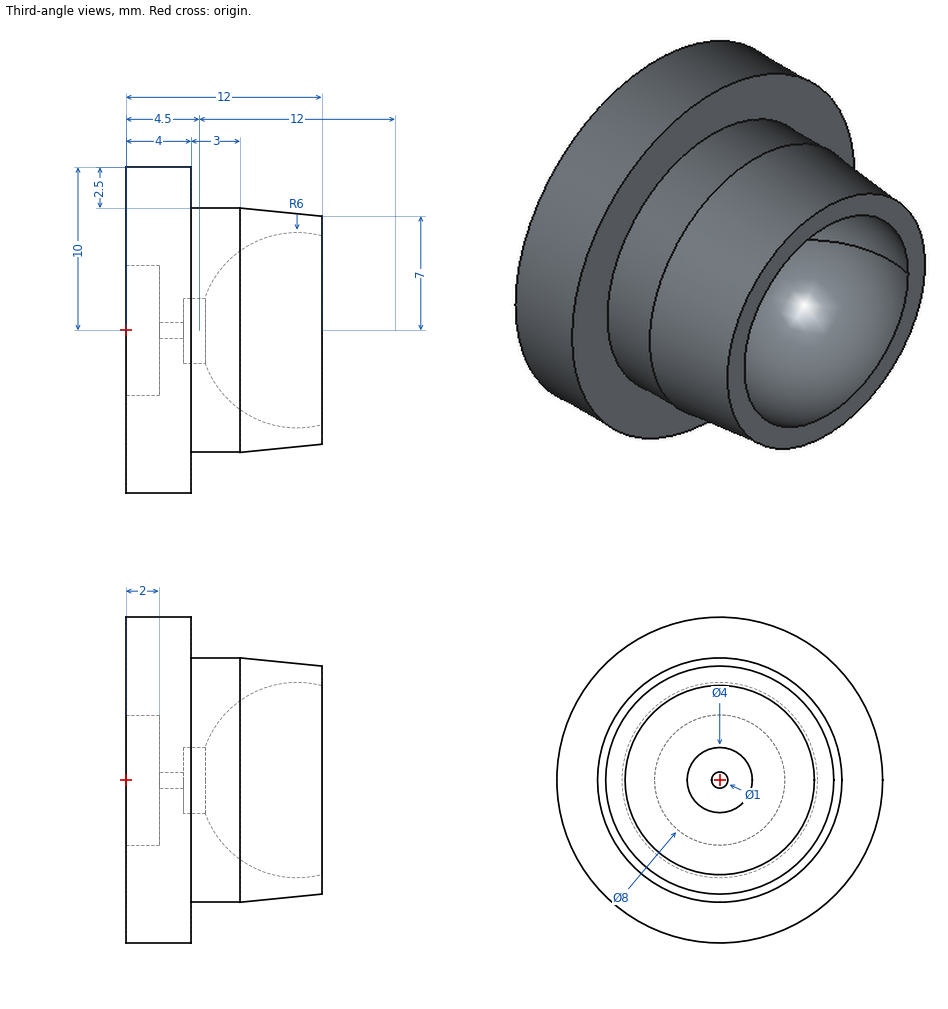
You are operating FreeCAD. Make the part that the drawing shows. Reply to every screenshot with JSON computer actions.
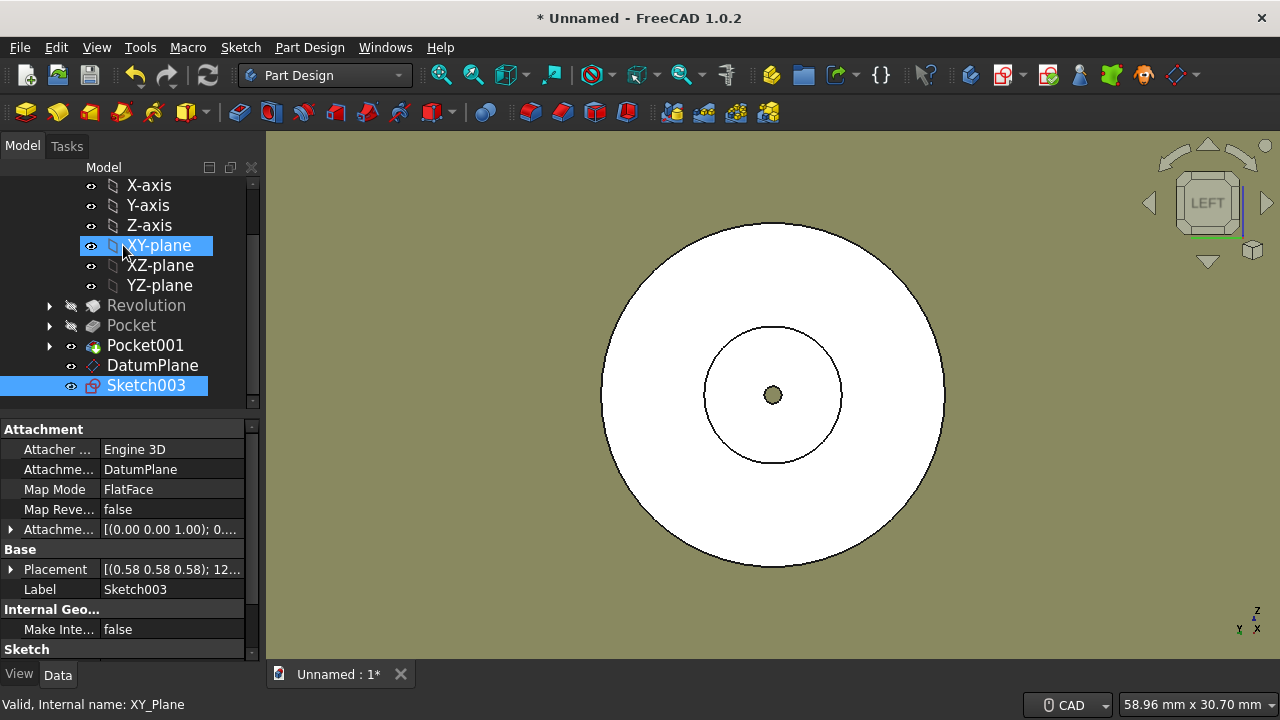
{"action": "left_click", "coordinate": [240, 112]}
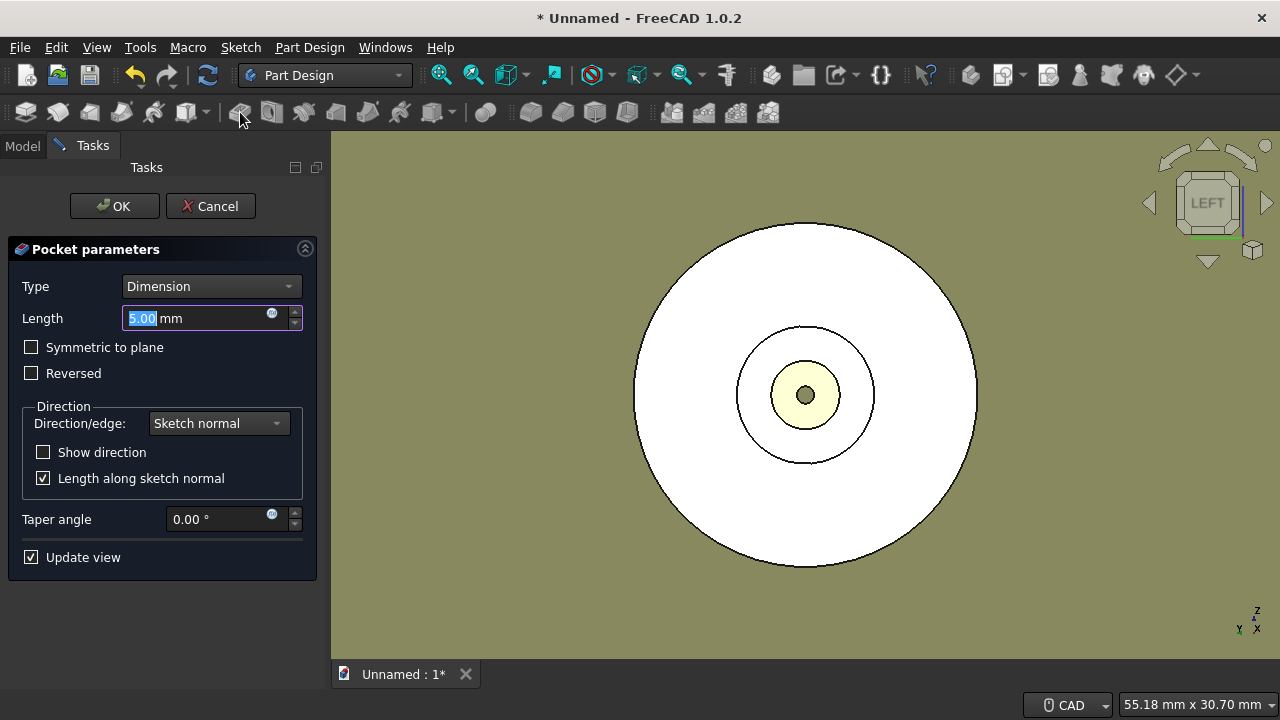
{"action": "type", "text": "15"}
{"action": "key", "text": "Tab"}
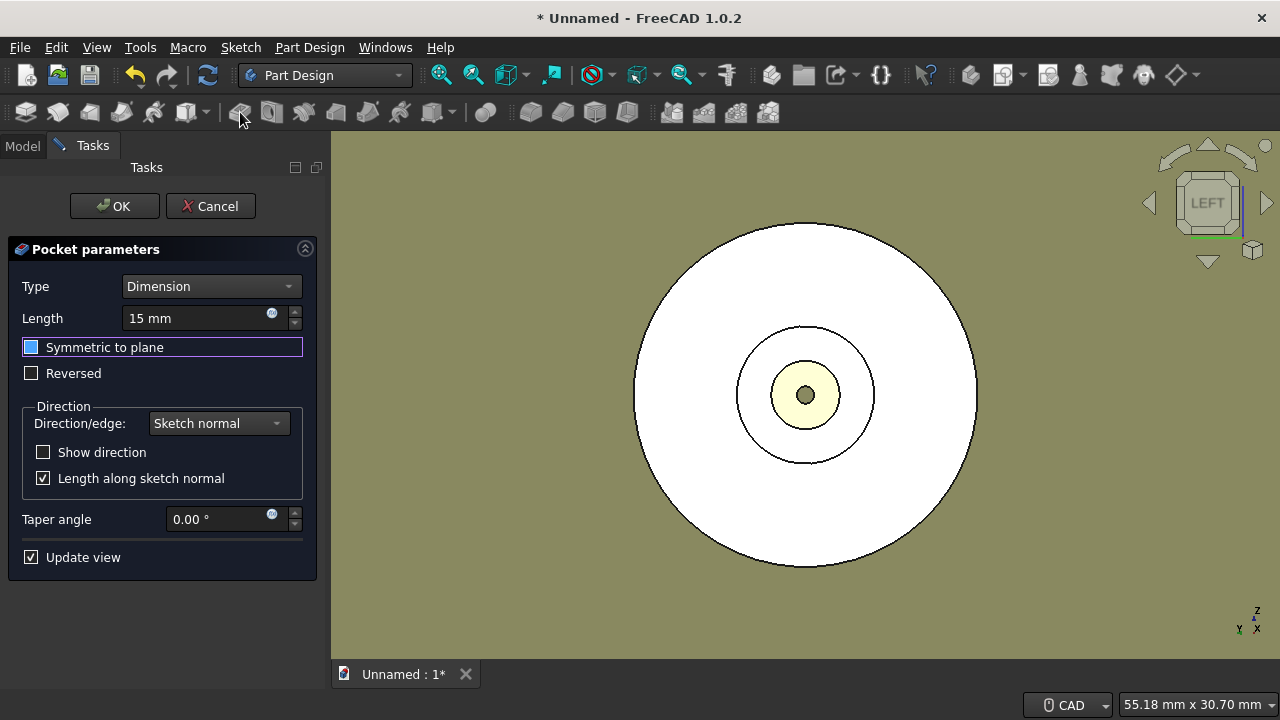
{"action": "left_click", "coordinate": [30, 373]}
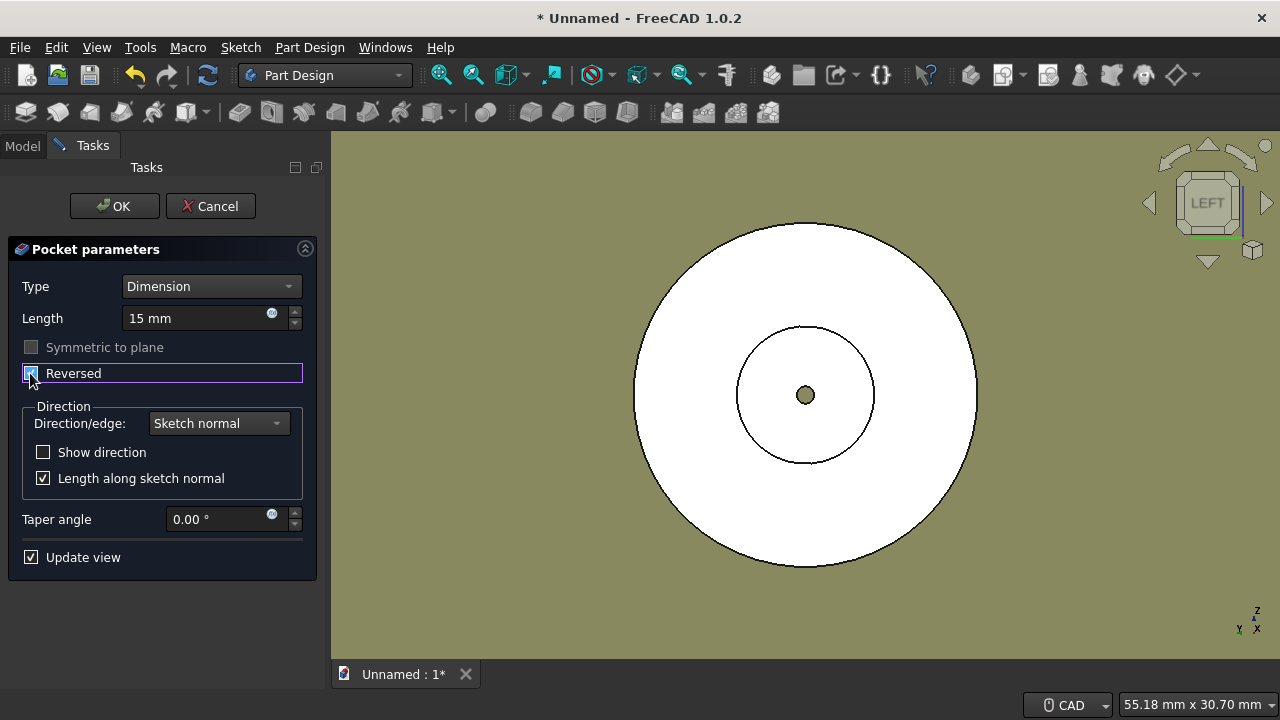
{"action": "left_click", "coordinate": [115, 206]}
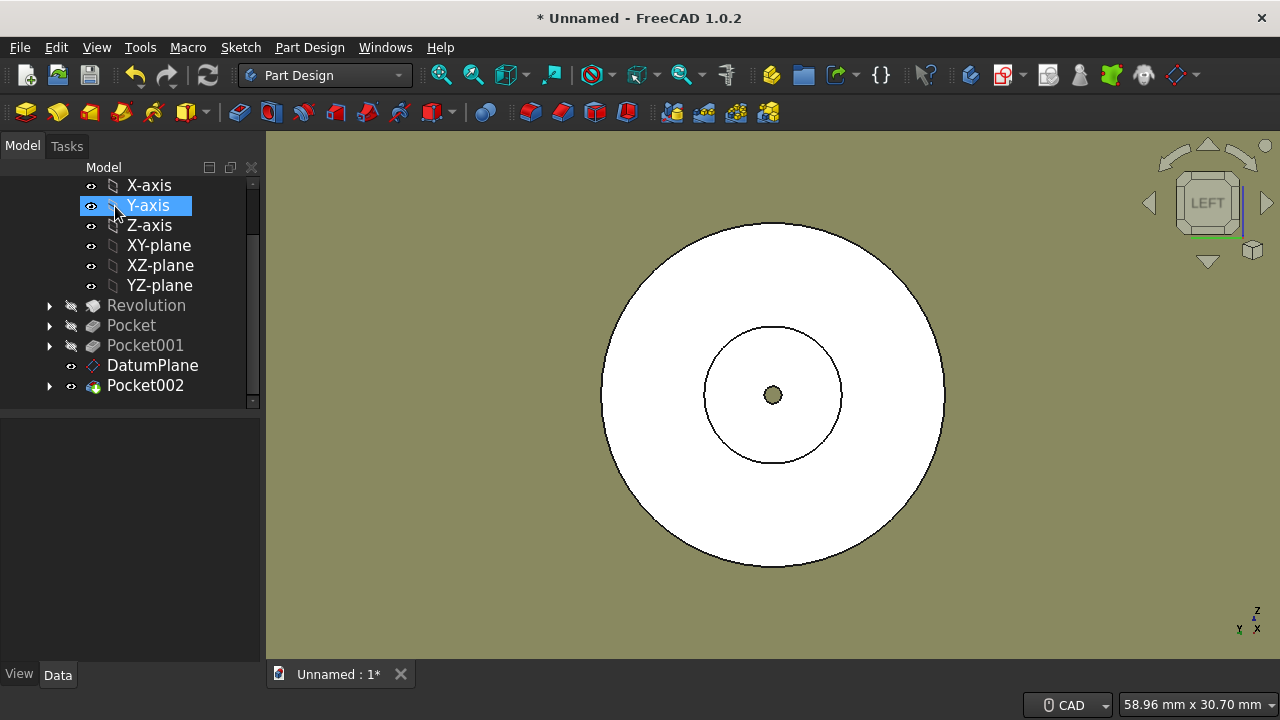
{"action": "left_click", "coordinate": [116, 366]}
{"action": "key", "text": "space"}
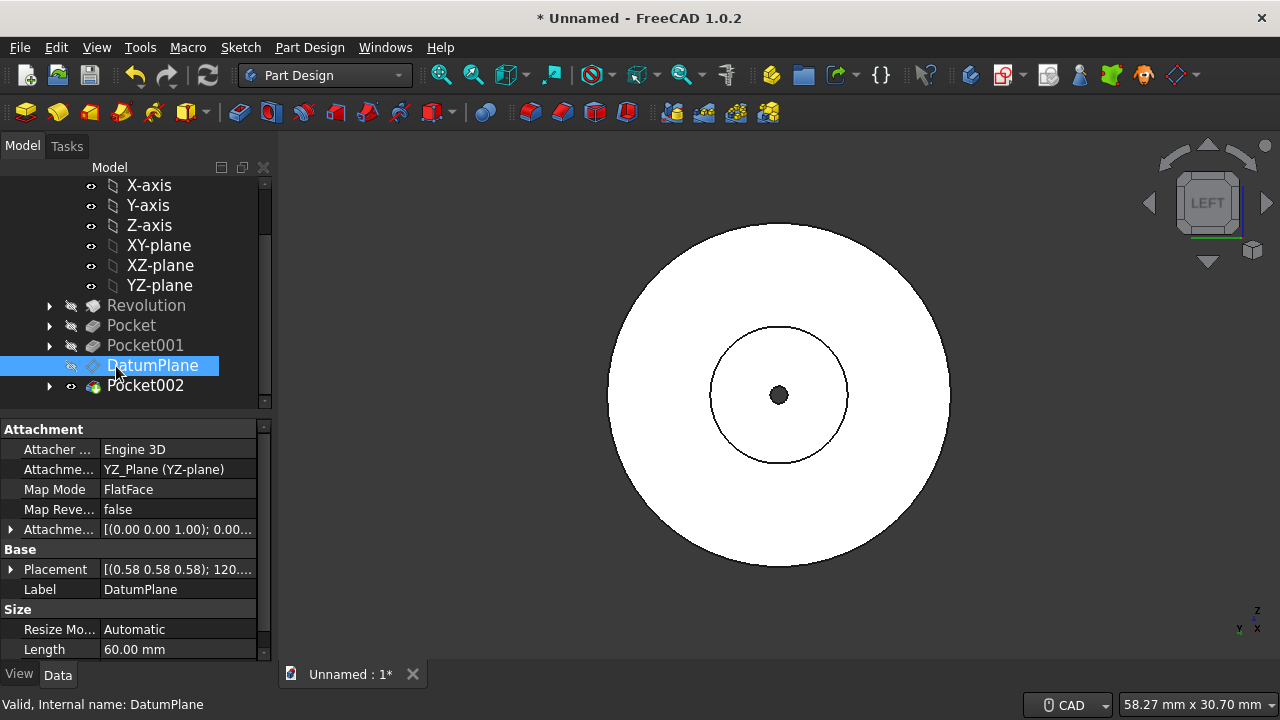
{"action": "left_click", "coordinate": [318, 619]}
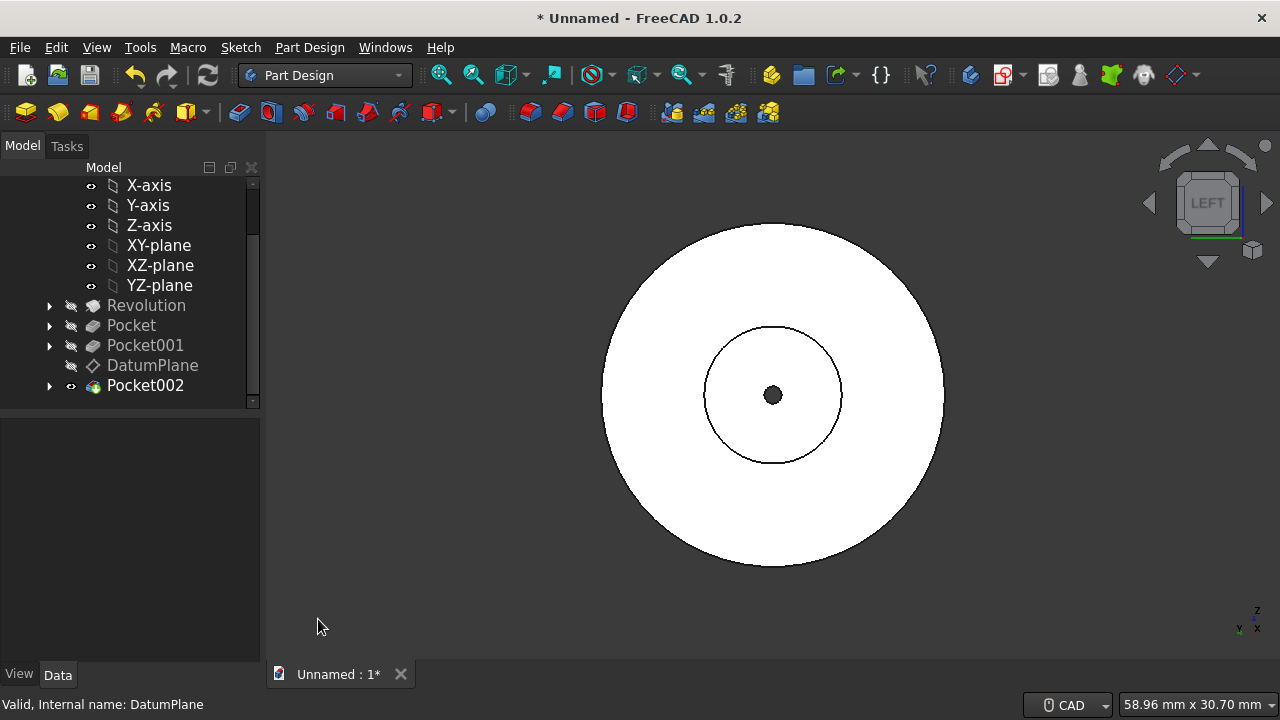
{"action": "left_click", "coordinate": [1004, 76]}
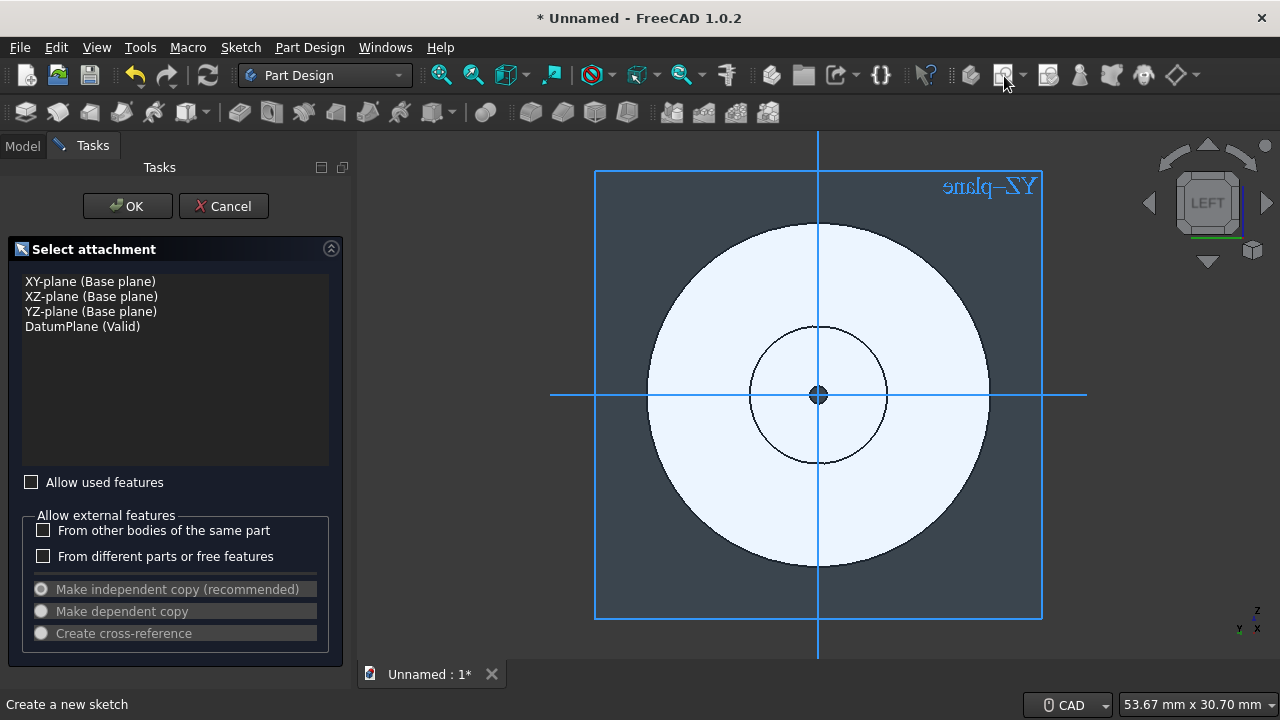
{"action": "left_click", "coordinate": [82, 282]}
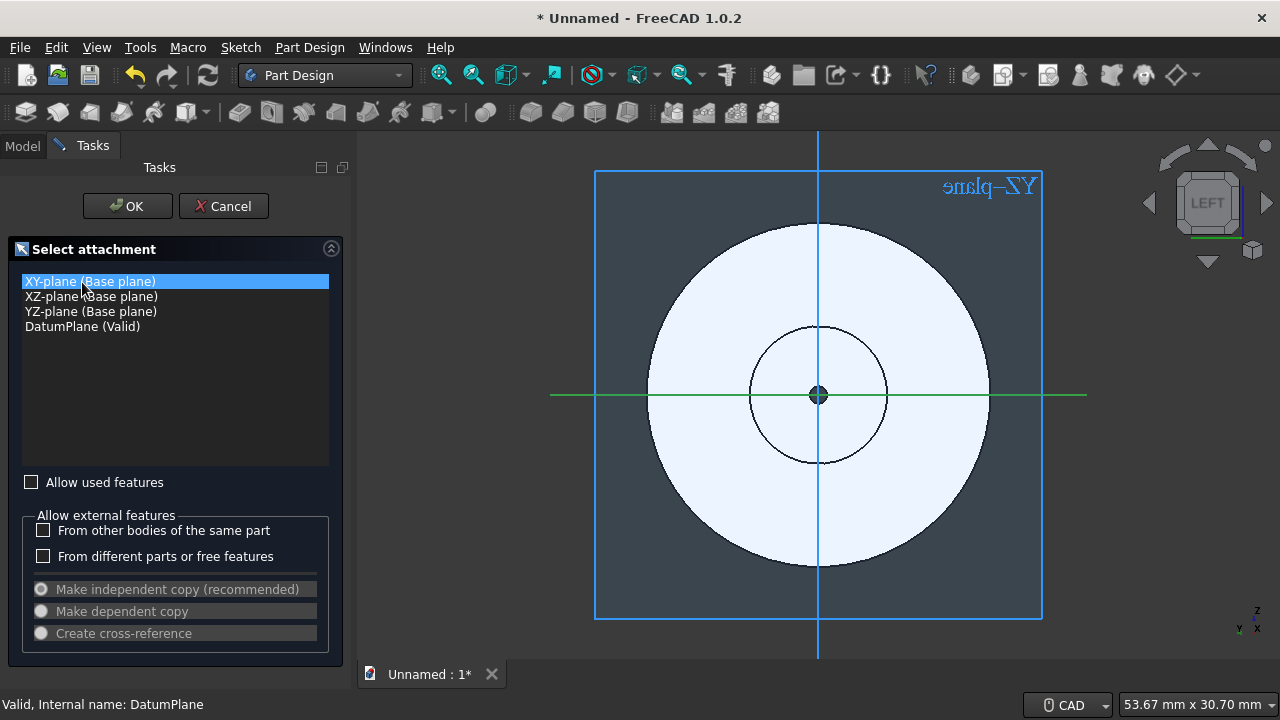
{"action": "left_click", "coordinate": [128, 206]}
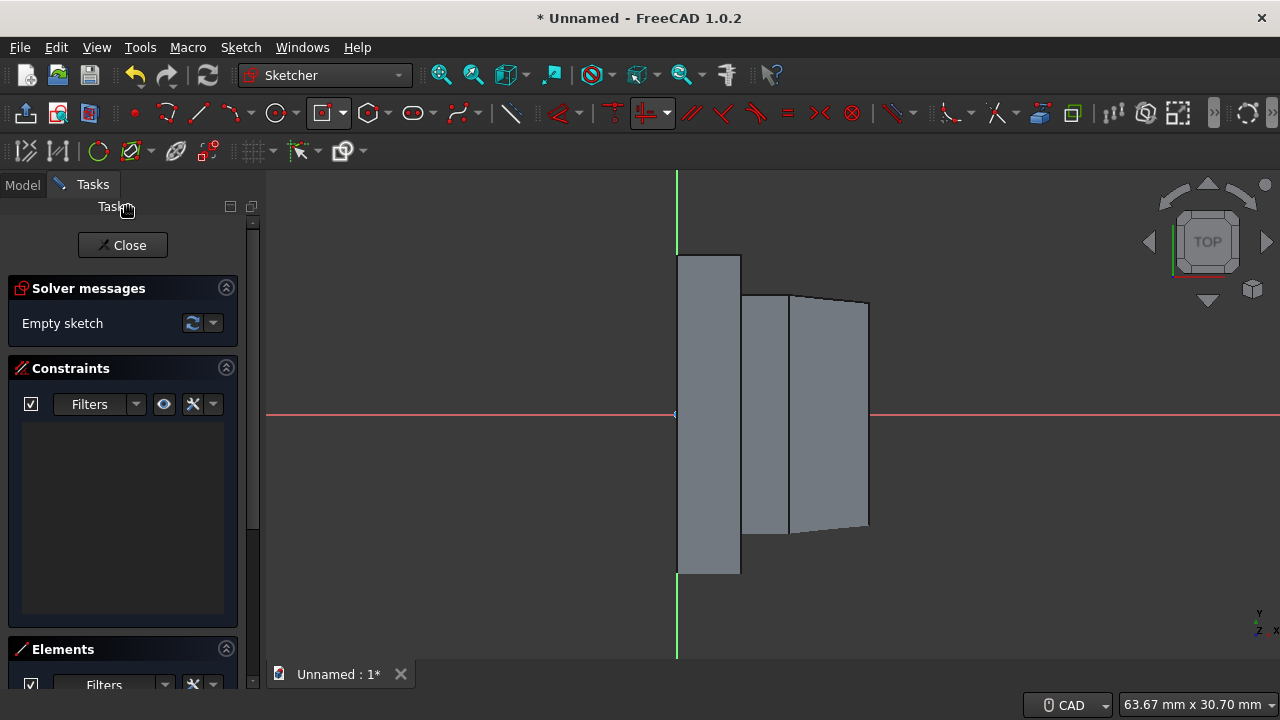
{"action": "left_click", "coordinate": [90, 114]}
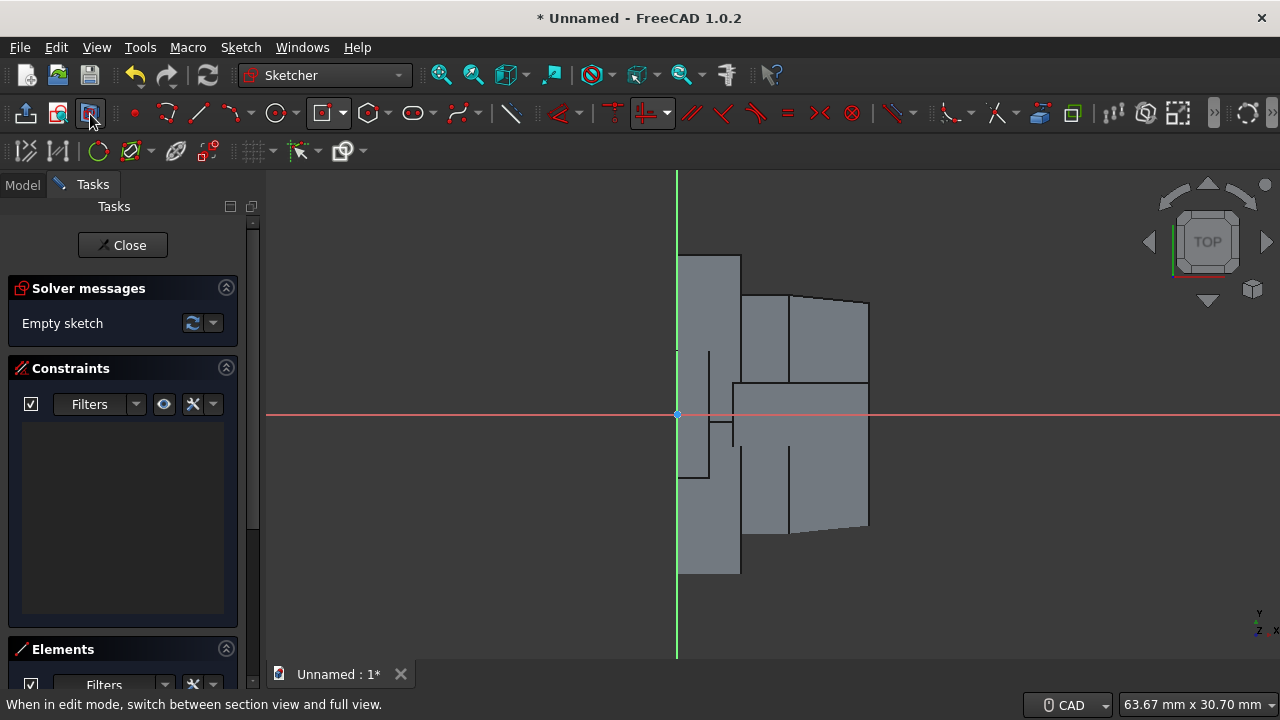
{"action": "scroll", "coordinate": [894, 328], "scroll_direction": "up", "scroll_amount": 4}